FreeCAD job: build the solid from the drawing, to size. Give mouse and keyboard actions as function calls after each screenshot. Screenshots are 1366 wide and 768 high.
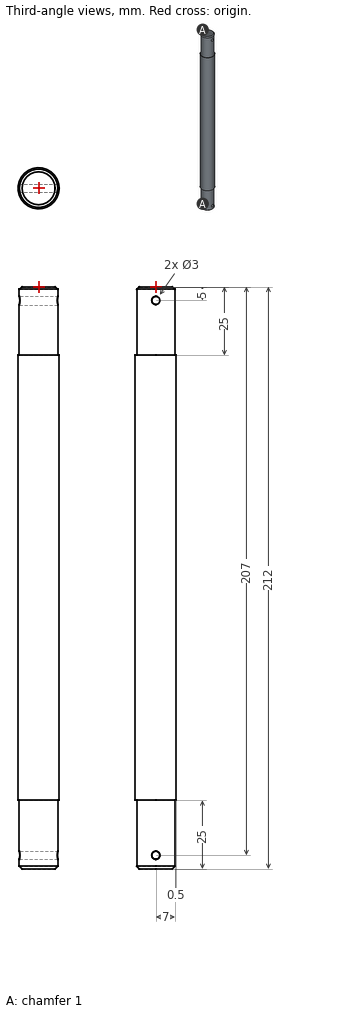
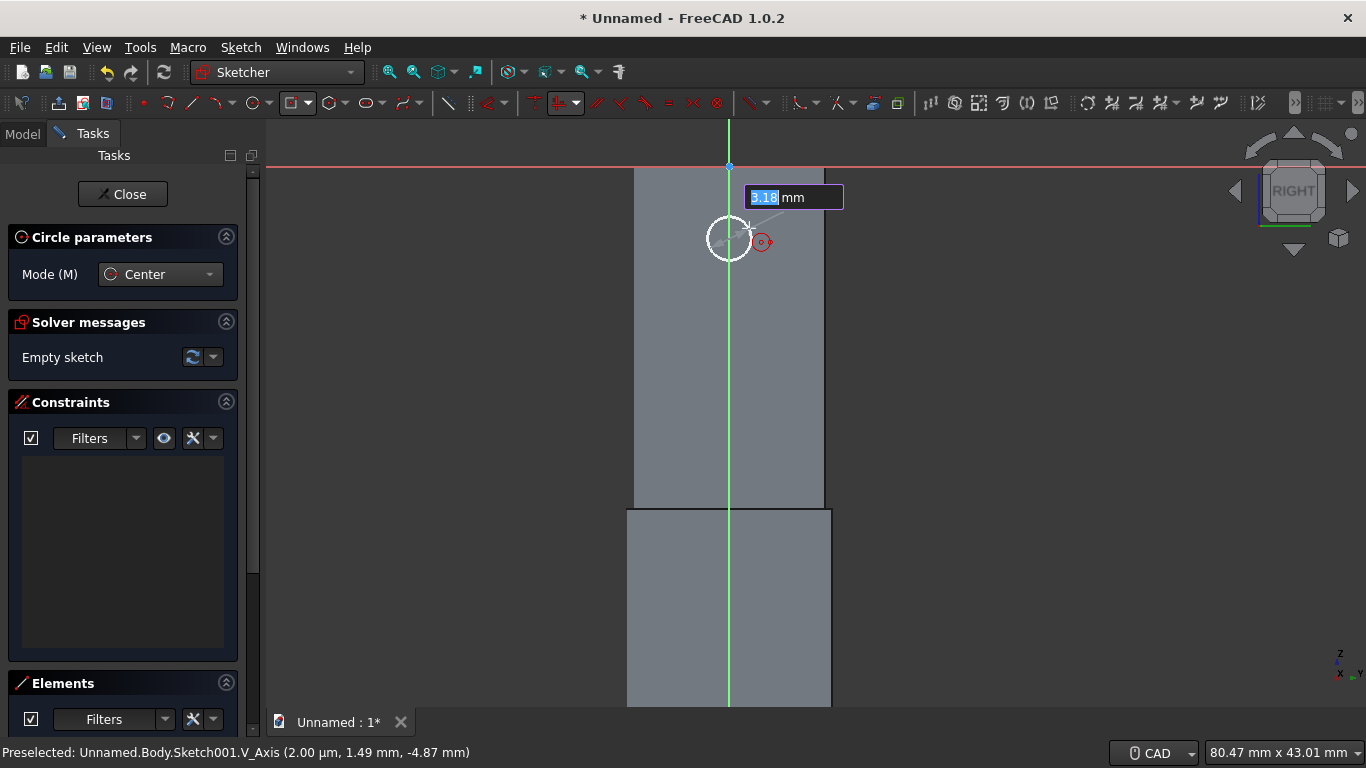
text(3)
key(Return)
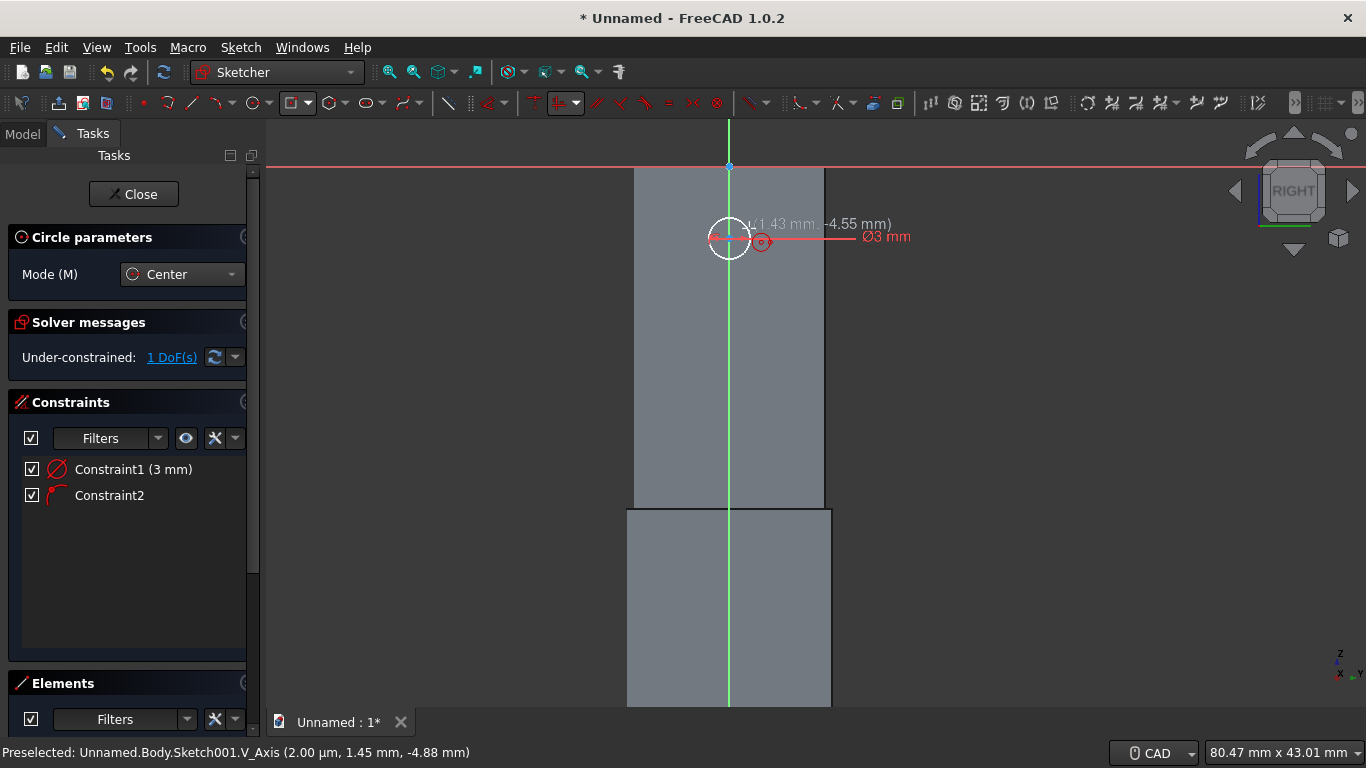
scroll(750, 228, down, 10)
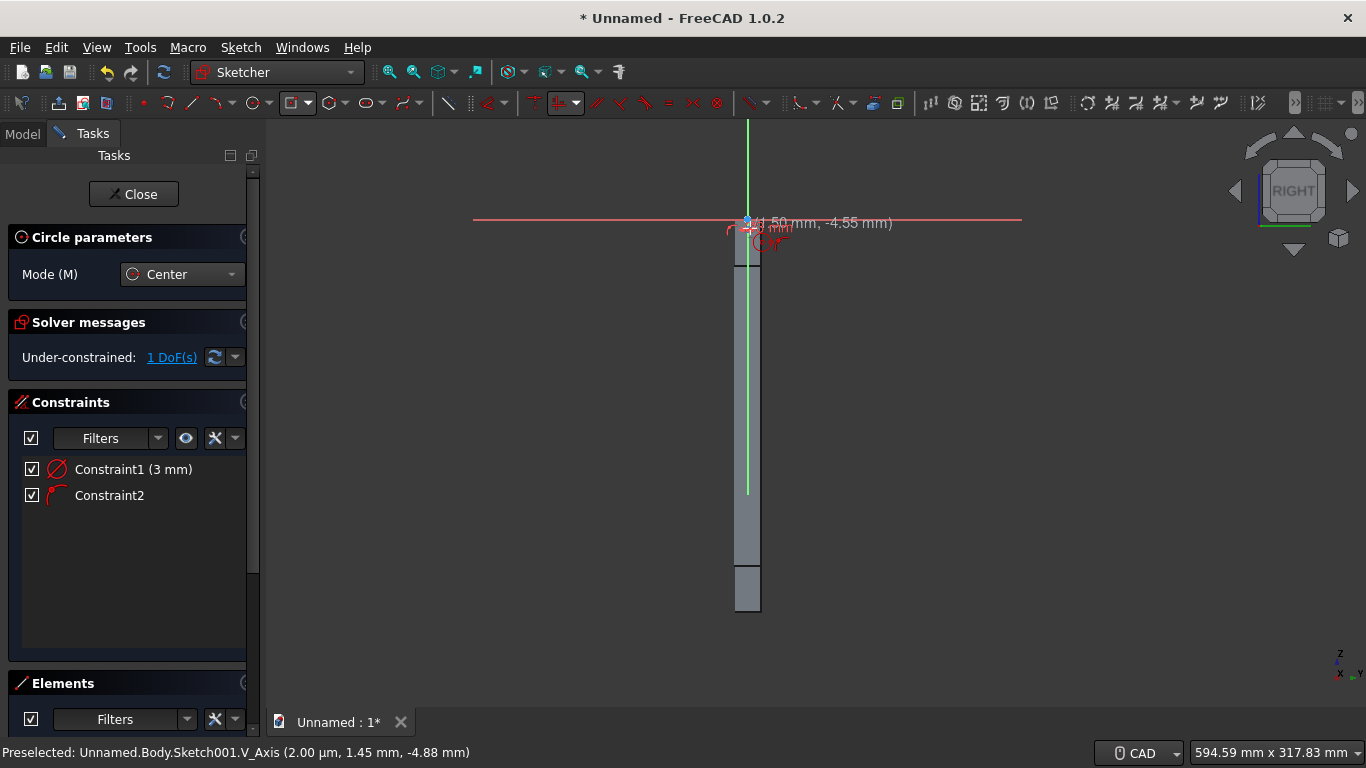
scroll(748, 603, up, 11)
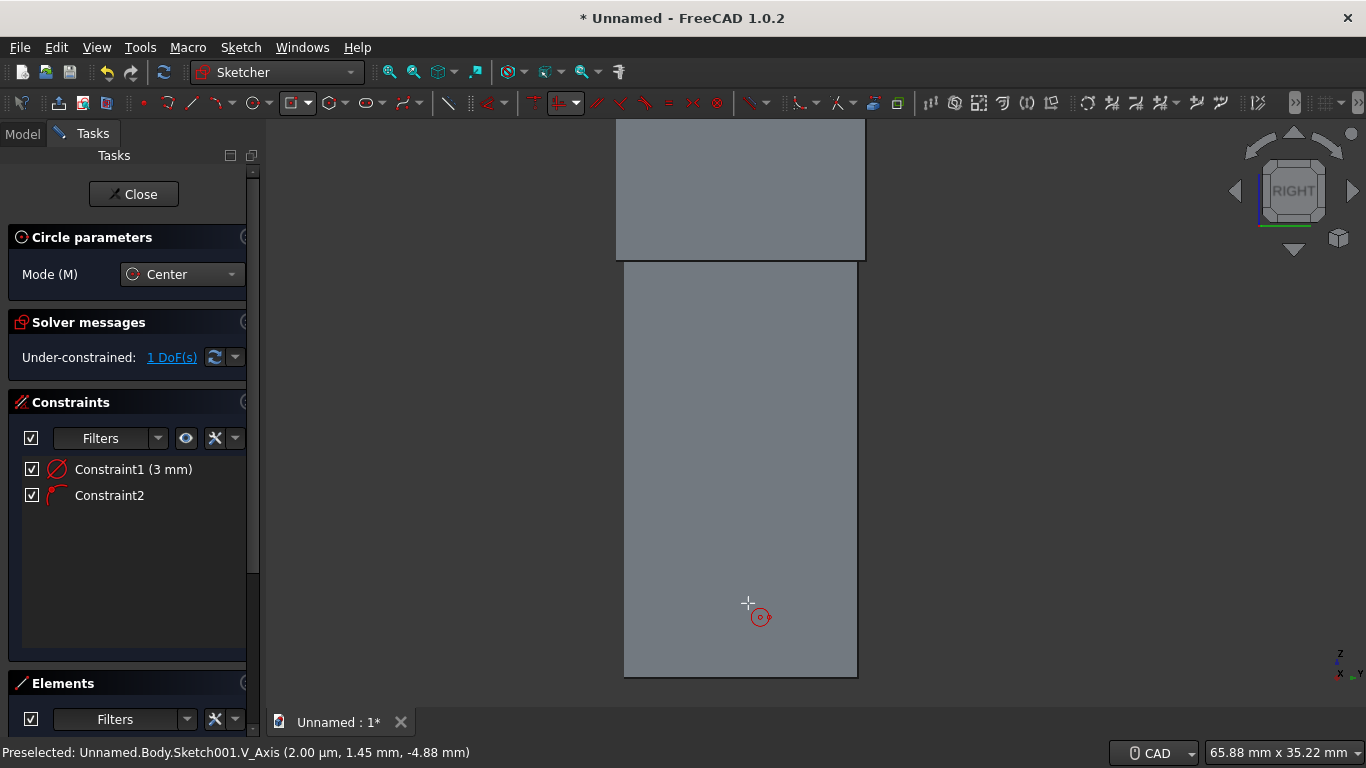
scroll(748, 604, down, 11)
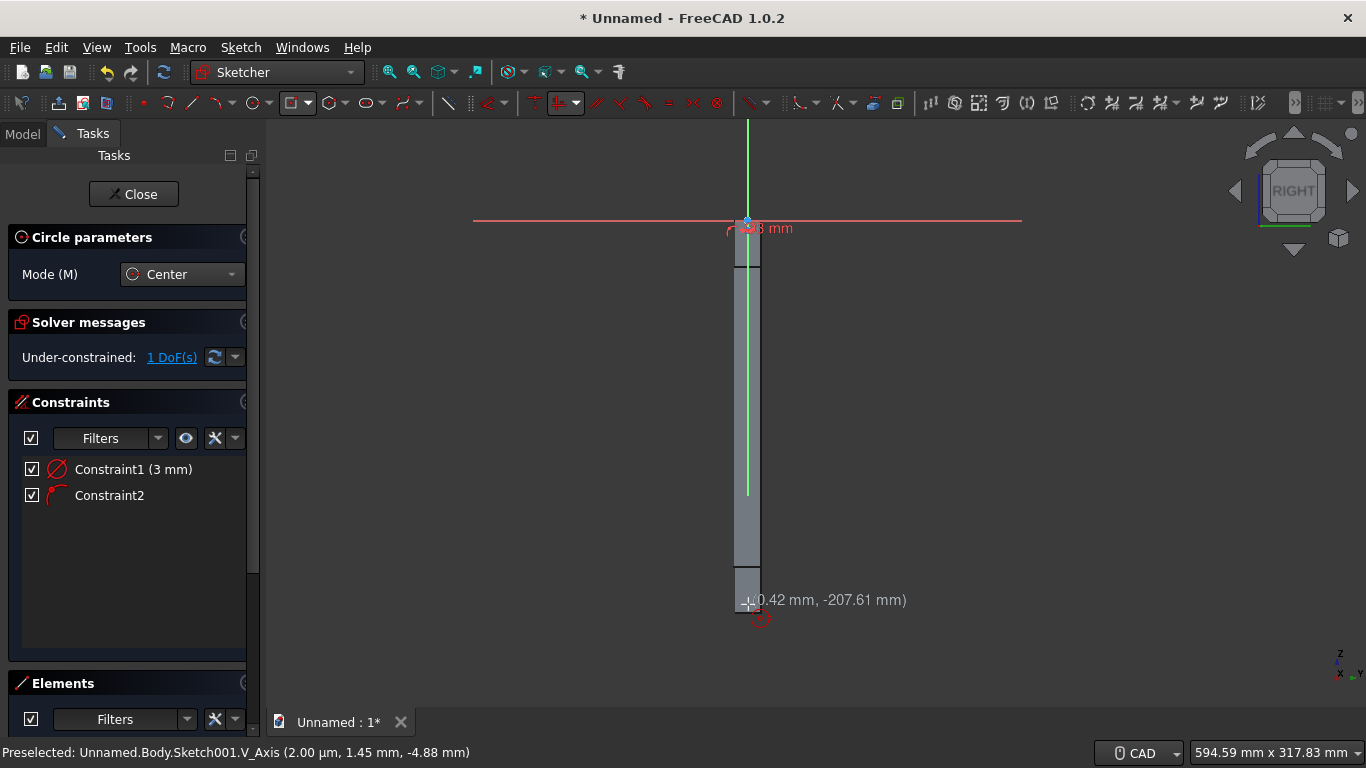
click(748, 604)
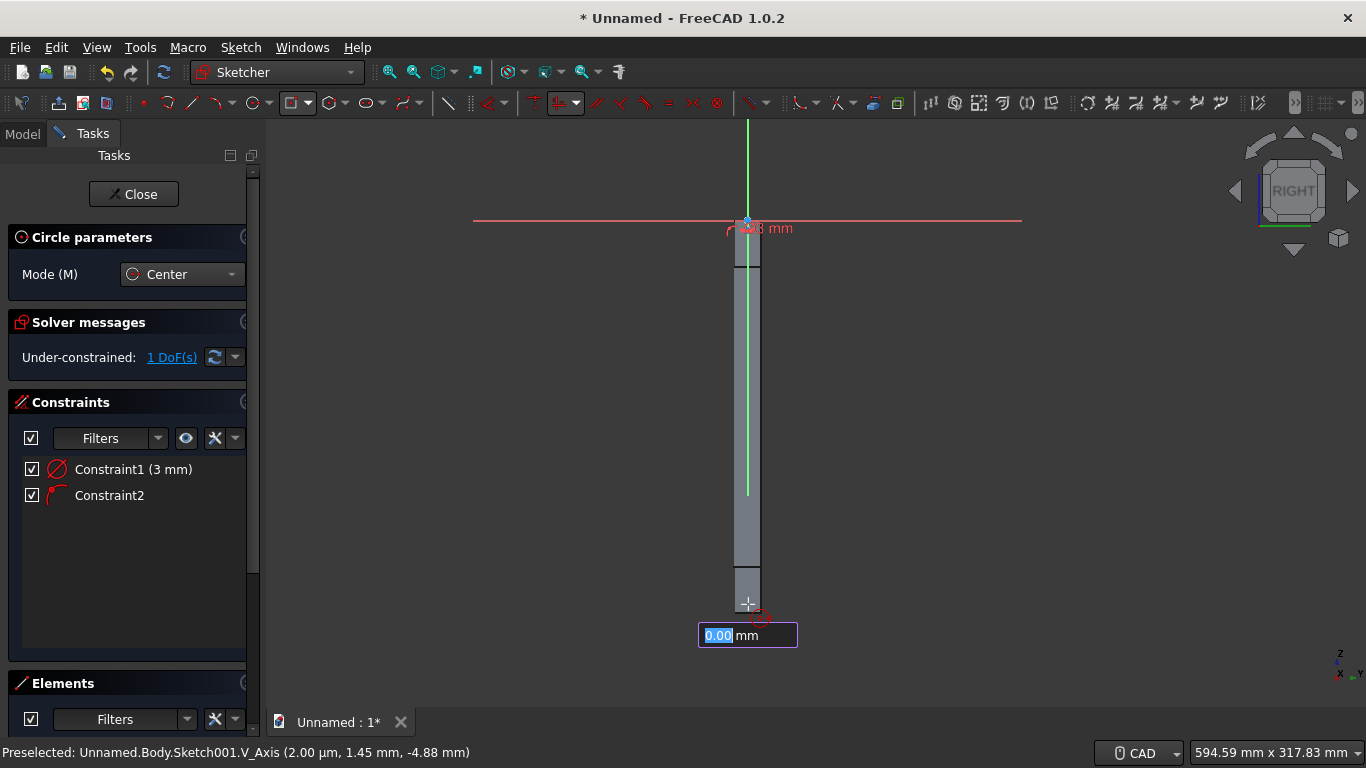
scroll(750, 603, up, 10)
move(749, 596)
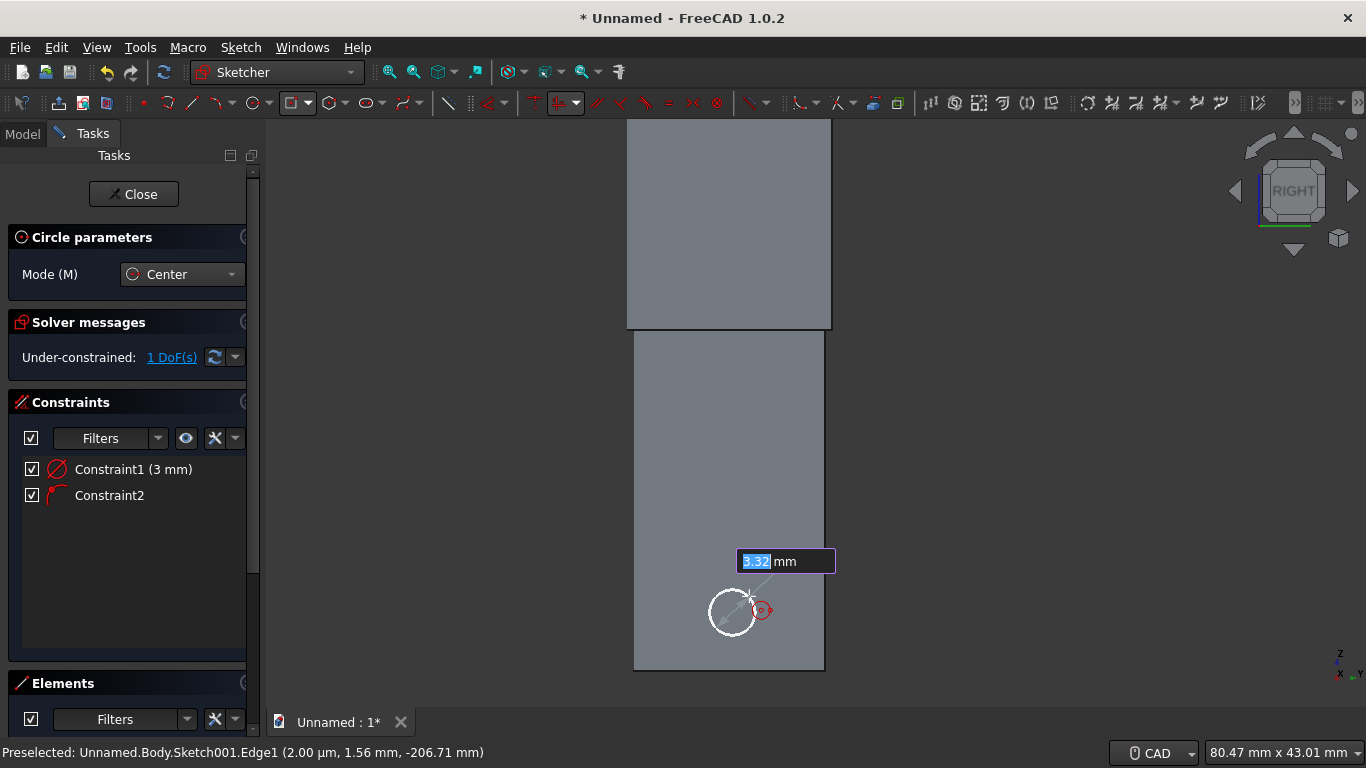
text(3)
key(Return)
key(Escape)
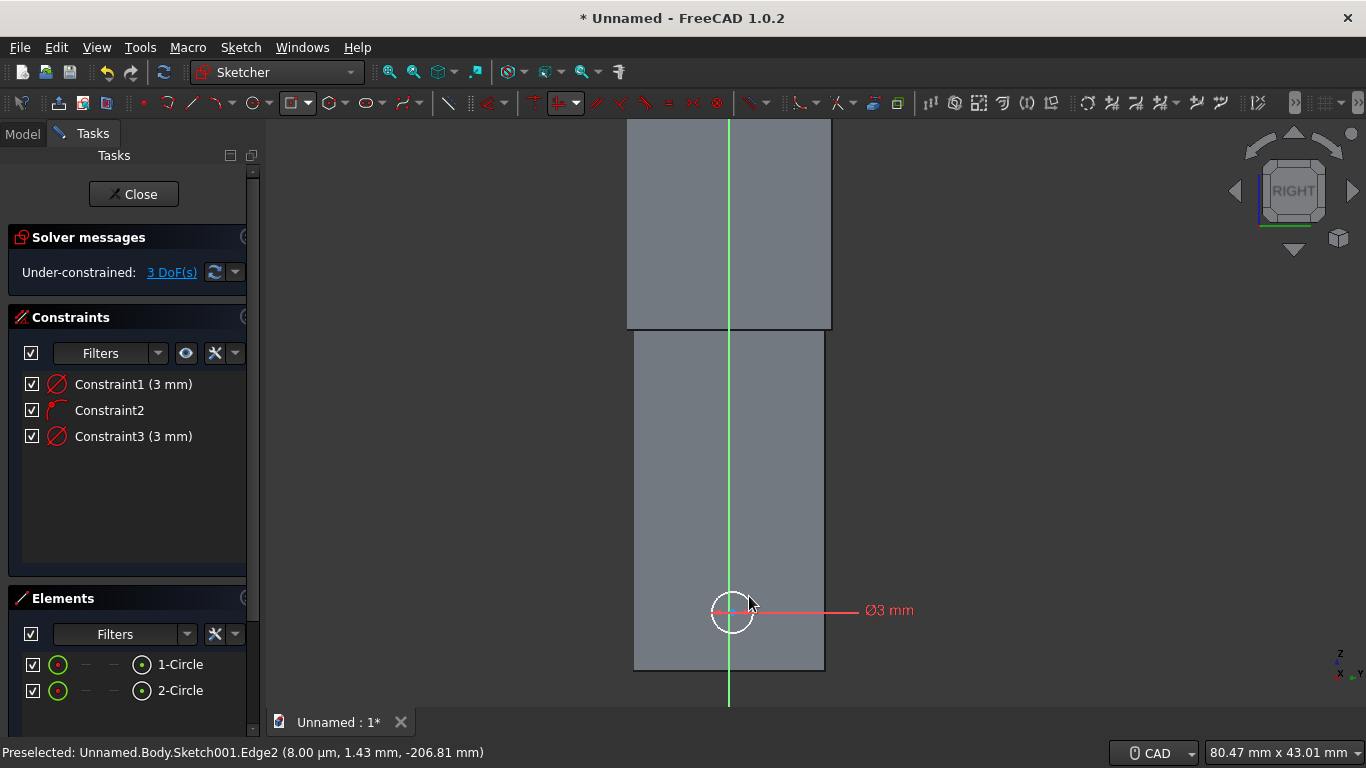
scroll(750, 603, down, 10)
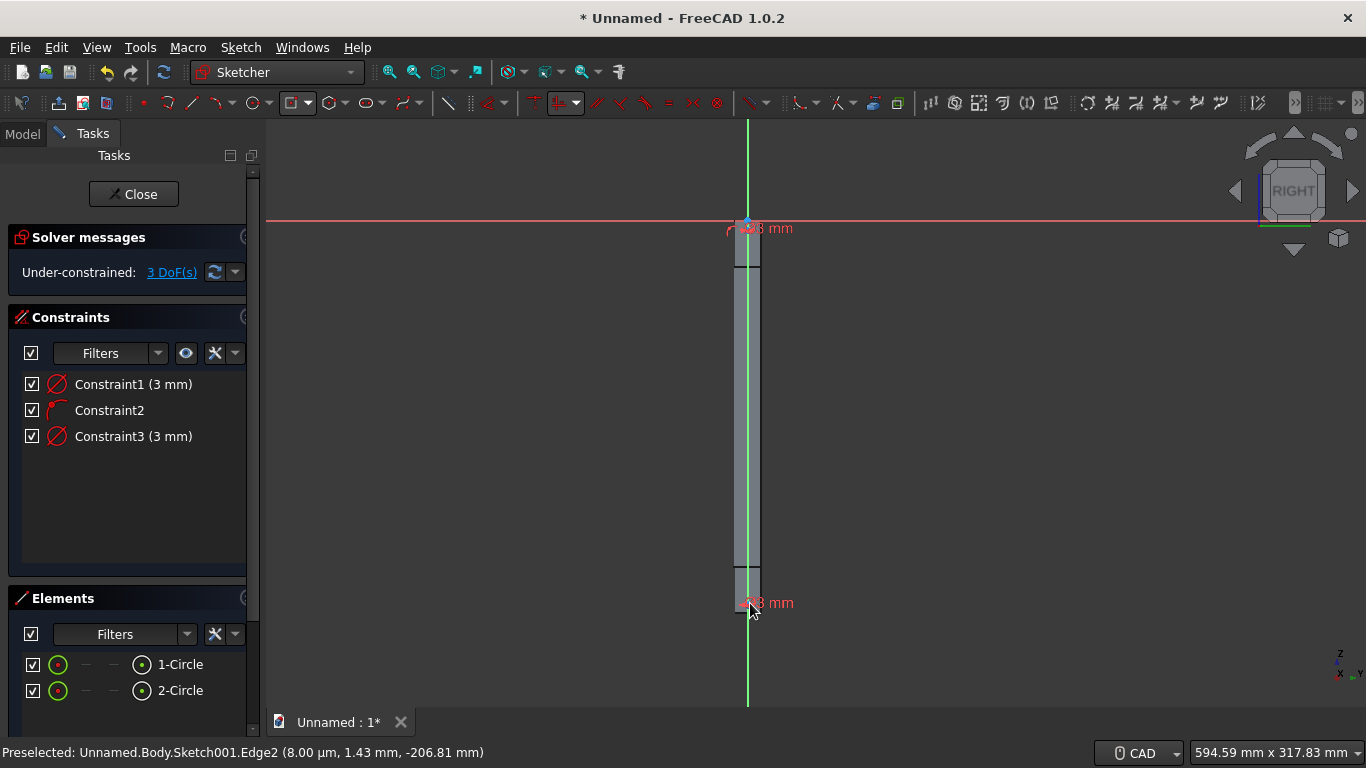
click(748, 605)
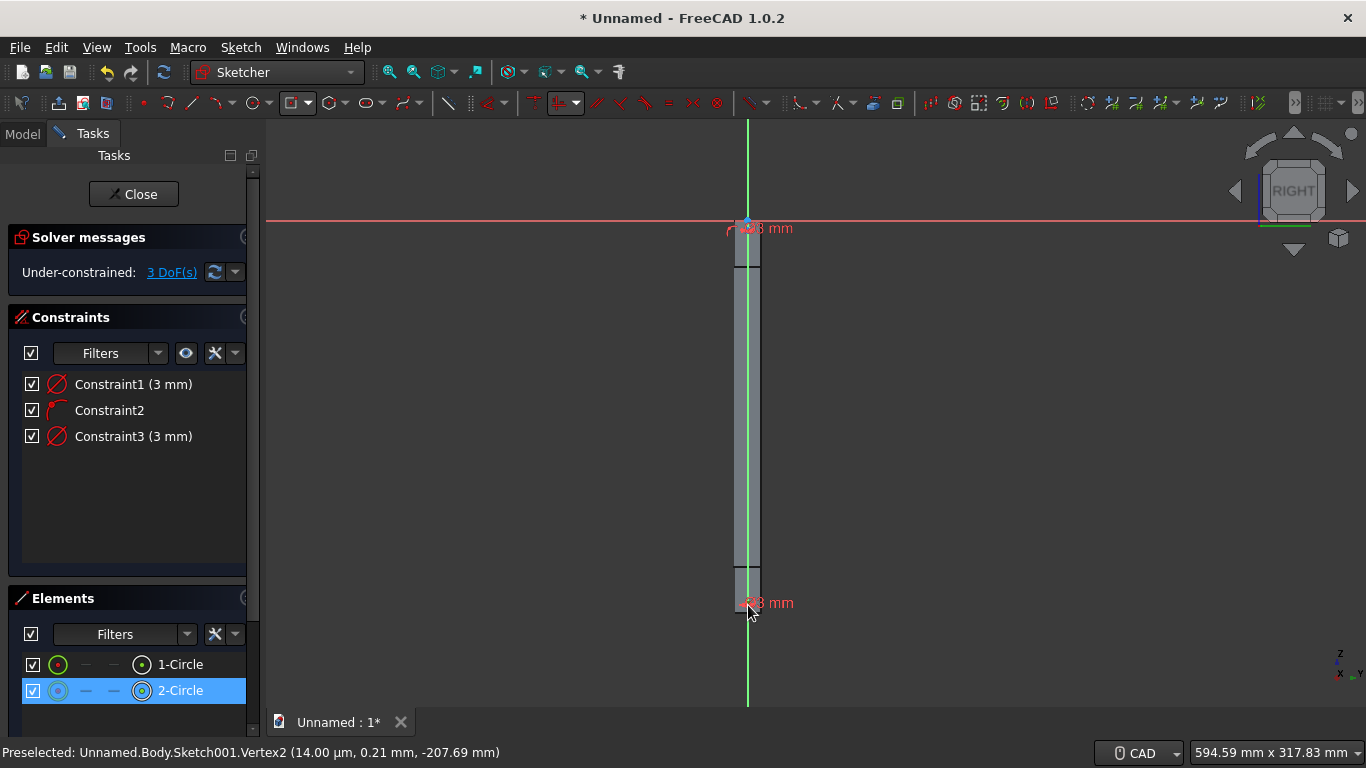
click(748, 641)